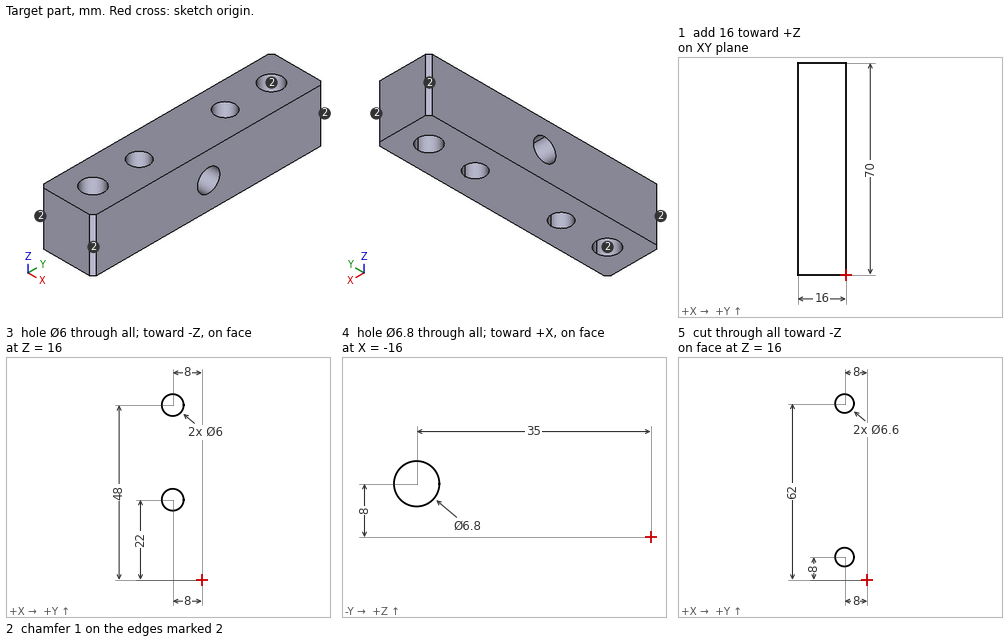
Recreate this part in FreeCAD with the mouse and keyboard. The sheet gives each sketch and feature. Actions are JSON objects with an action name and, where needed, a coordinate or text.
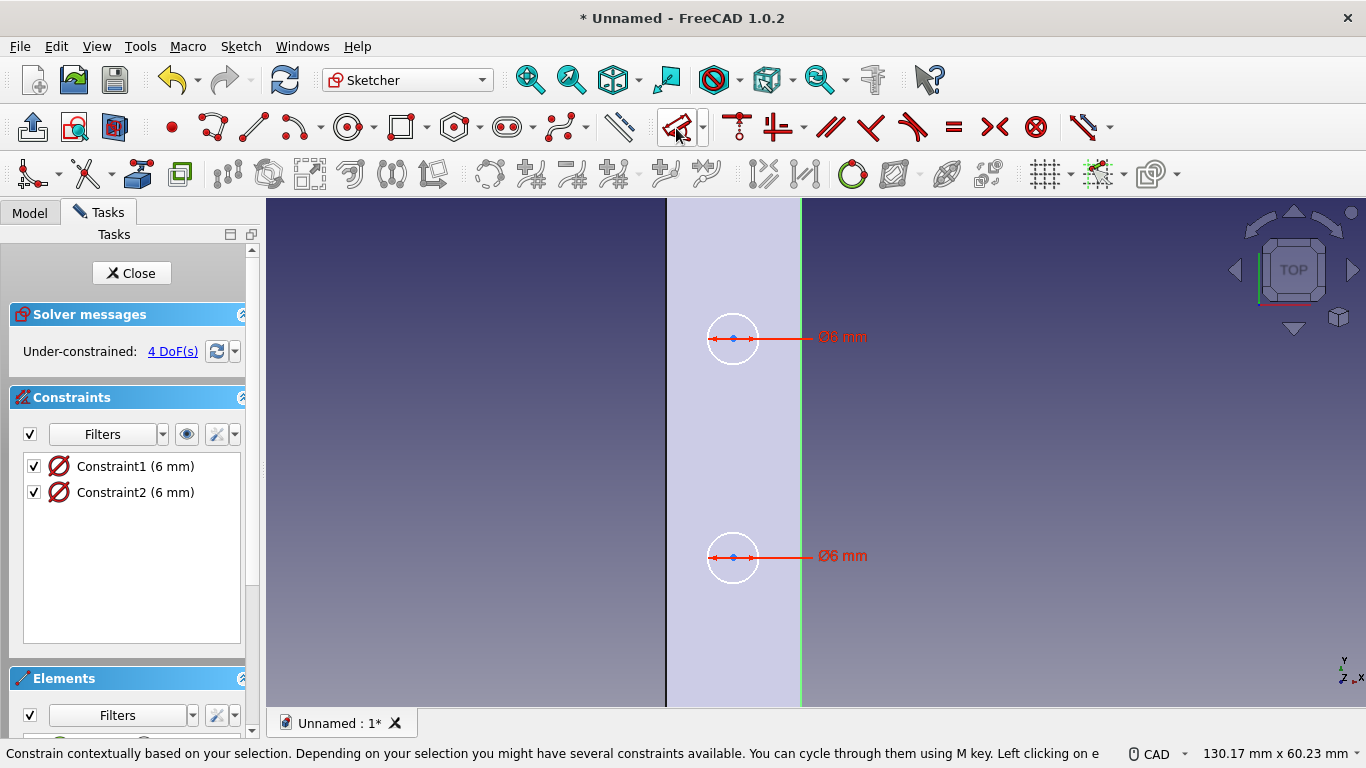
{"action": "left_click", "coordinate": [733, 339]}
{"action": "left_click", "coordinate": [767, 305]}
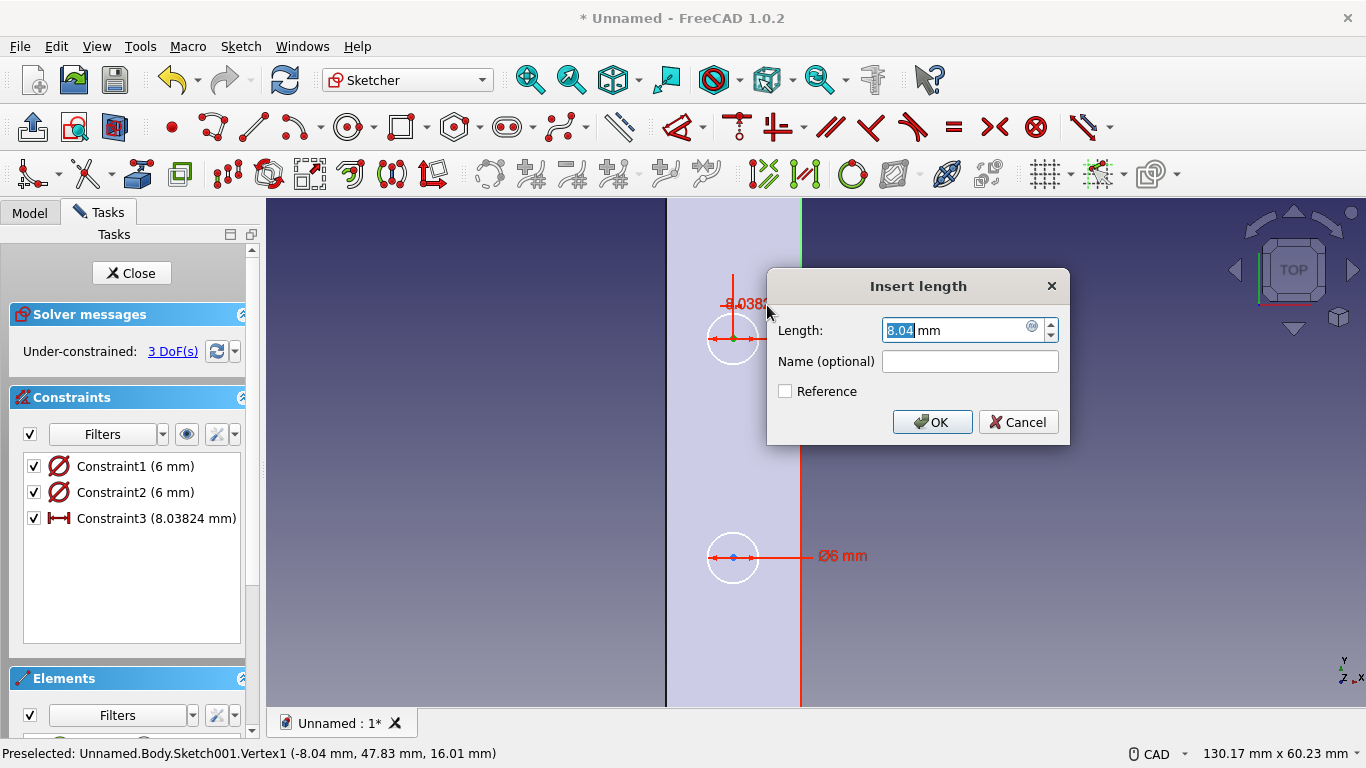
{"action": "type", "text": "8"}
{"action": "key", "text": "Return"}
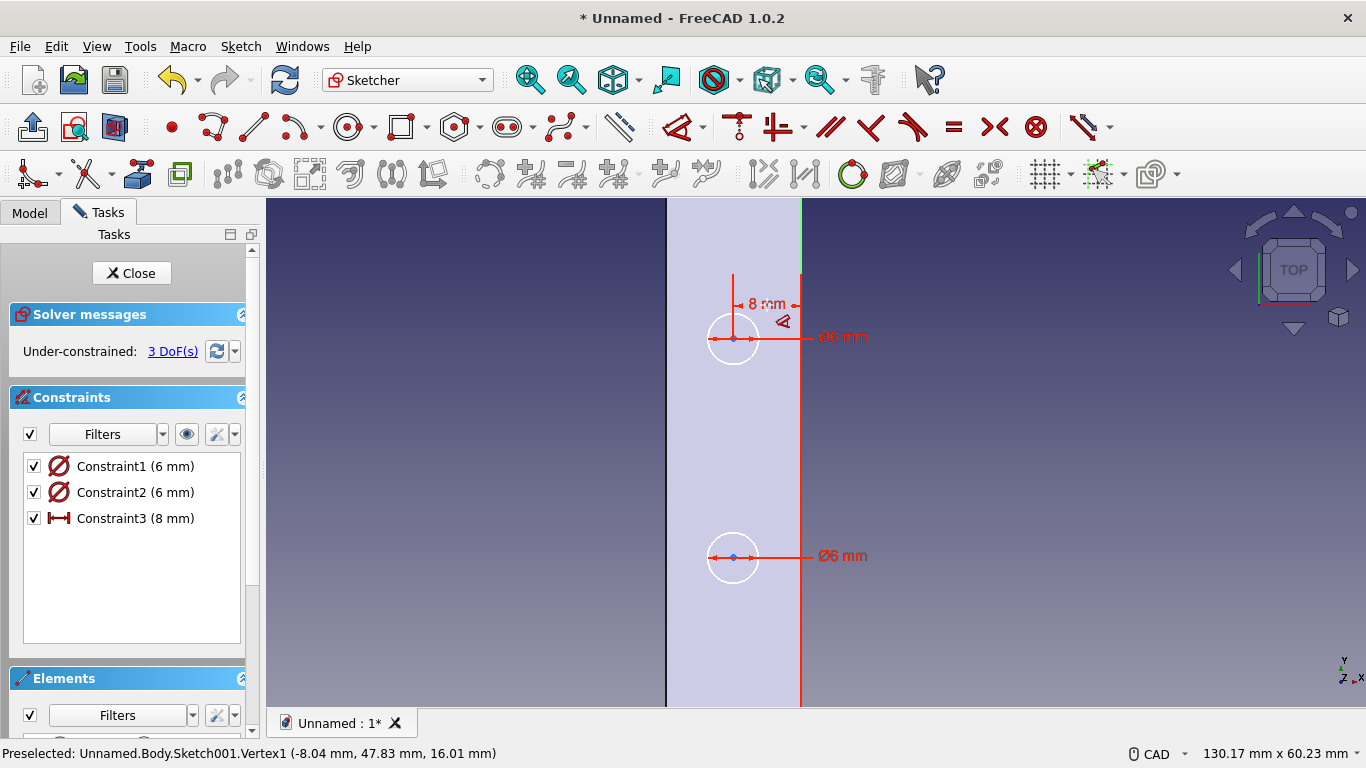
{"action": "left_click", "coordinate": [733, 558]}
{"action": "left_click", "coordinate": [767, 524]}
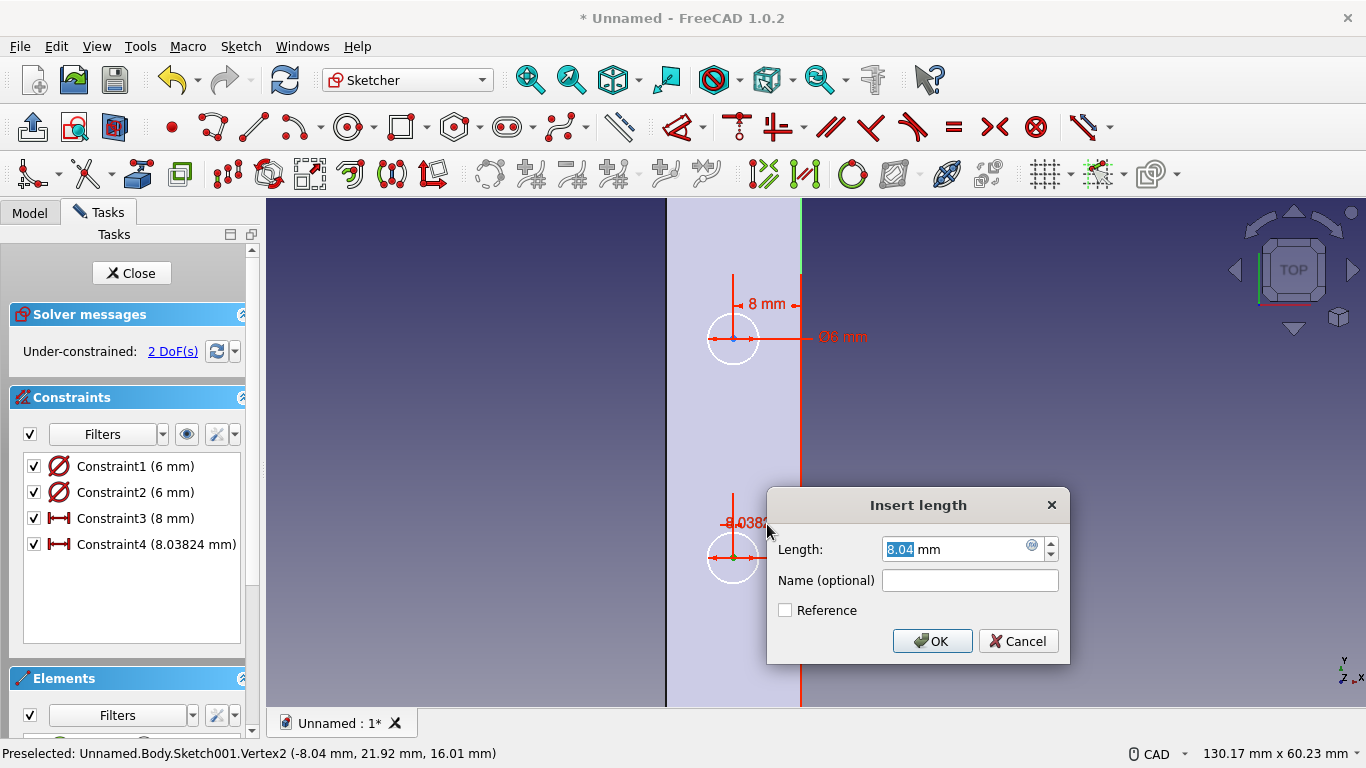
{"action": "type", "text": "8"}
{"action": "key", "text": "Return"}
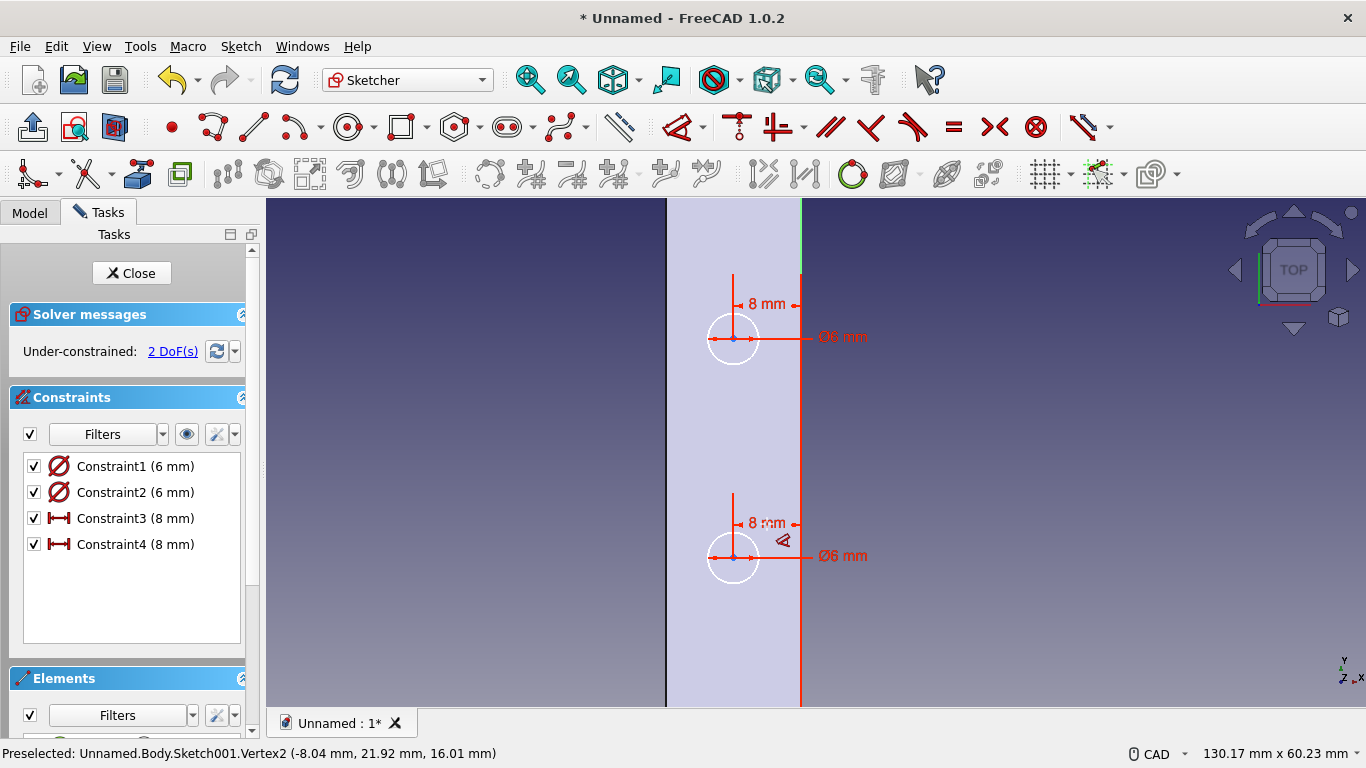
{"action": "left_click", "coordinate": [733, 339]}
{"action": "left_click", "coordinate": [835, 431]}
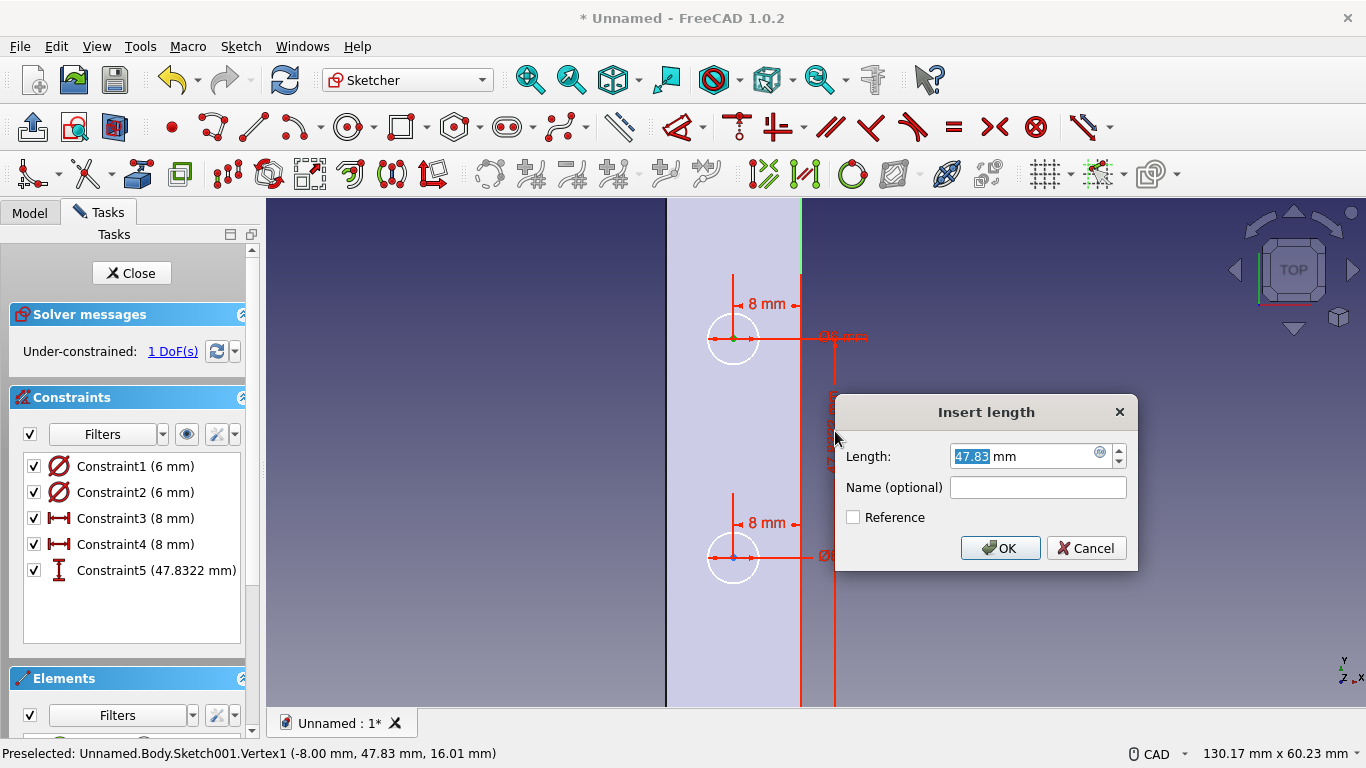
{"action": "type", "text": "48"}
{"action": "key", "text": "Return"}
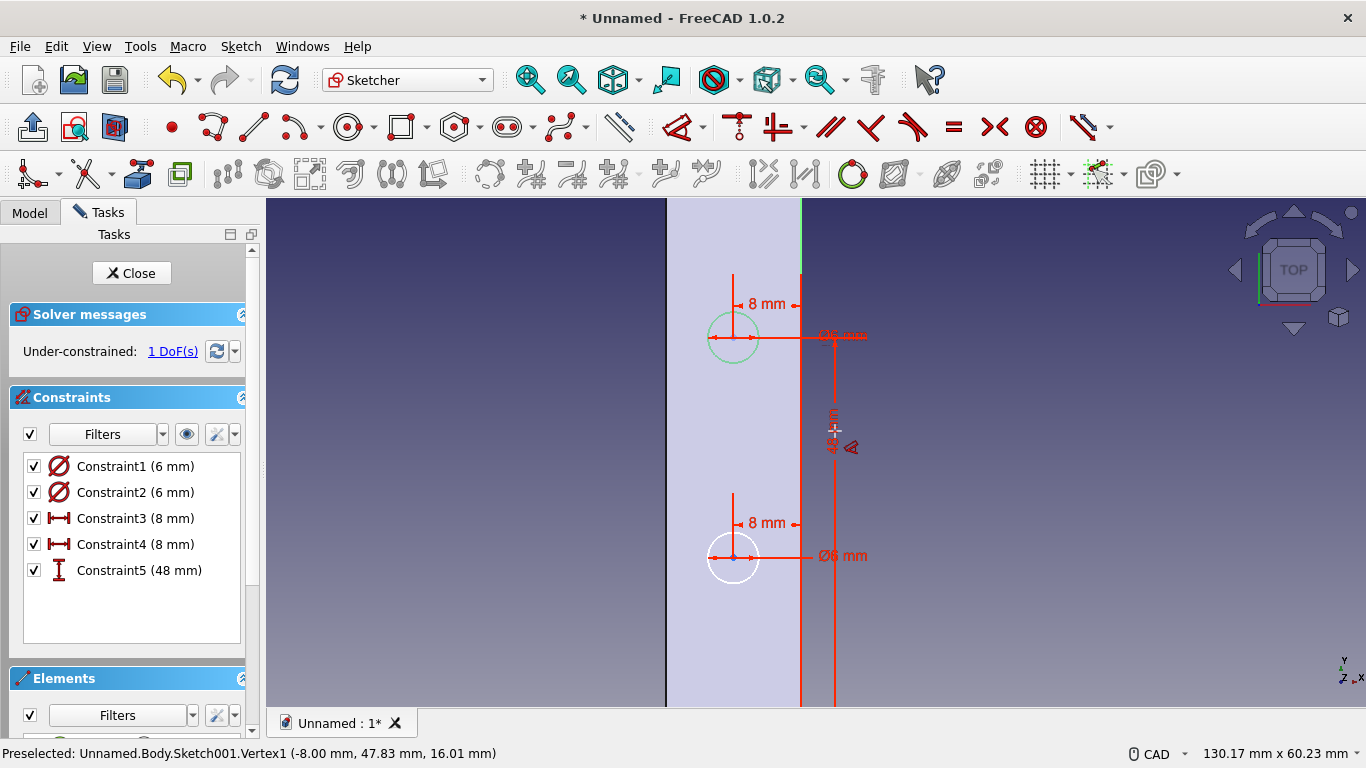
{"action": "left_click", "coordinate": [733, 558]}
{"action": "left_click", "coordinate": [835, 619]}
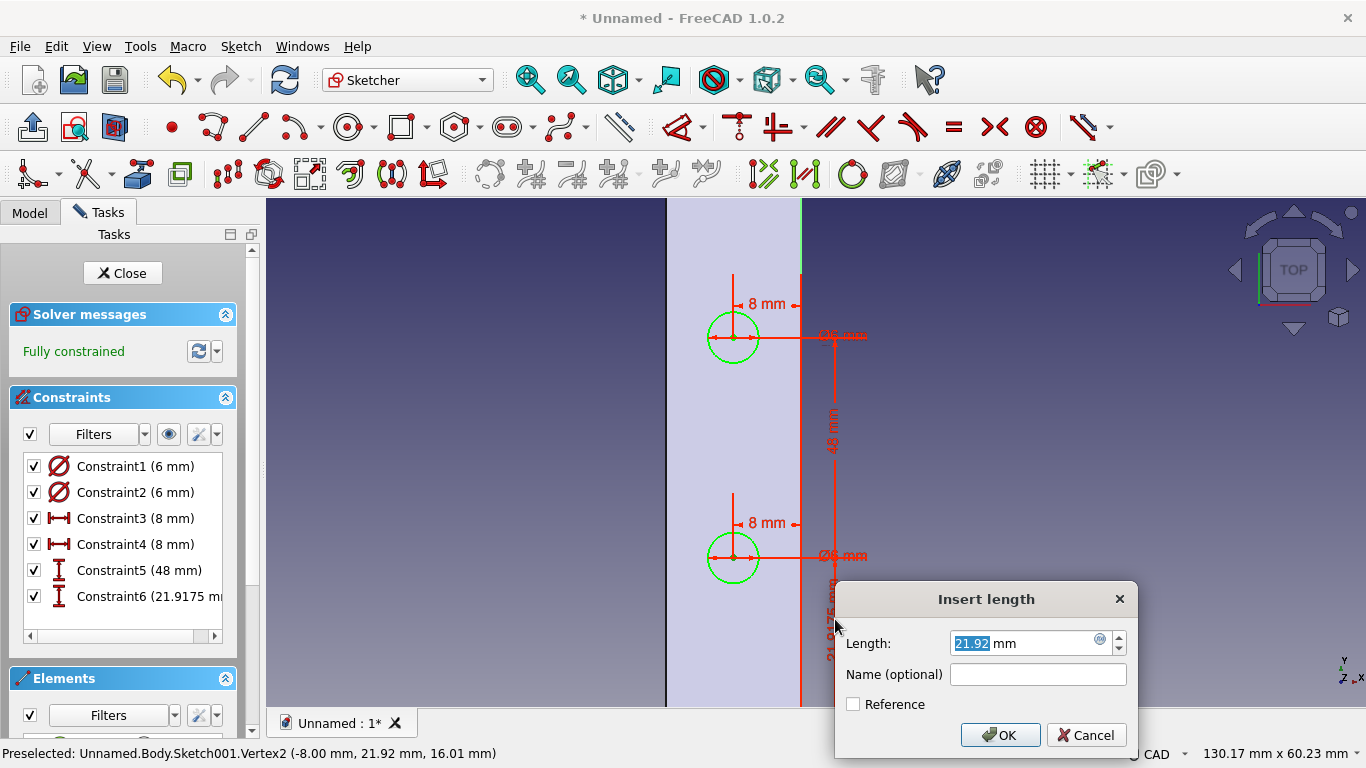
{"action": "type", "text": "22"}
{"action": "key", "text": "Return"}
{"action": "key", "text": "Escape"}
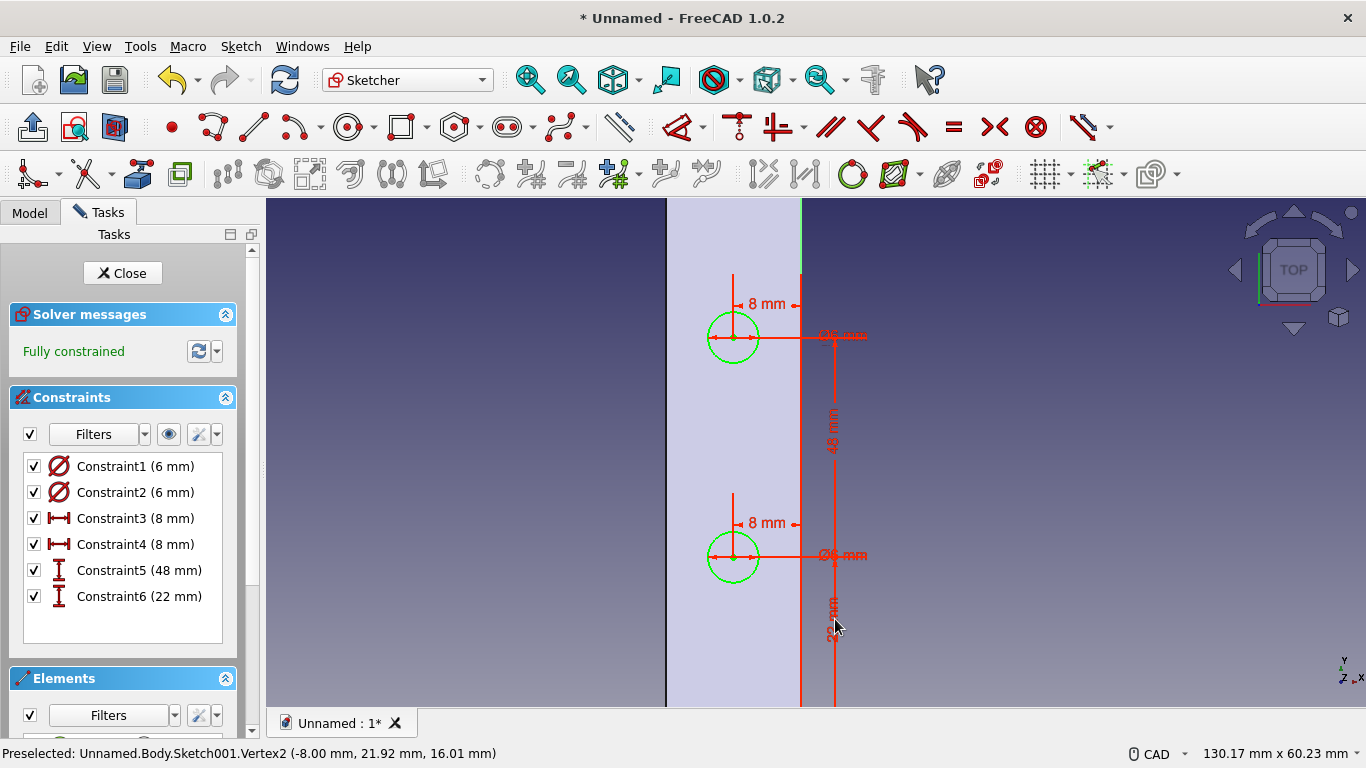
{"action": "left_click", "coordinate": [123, 273]}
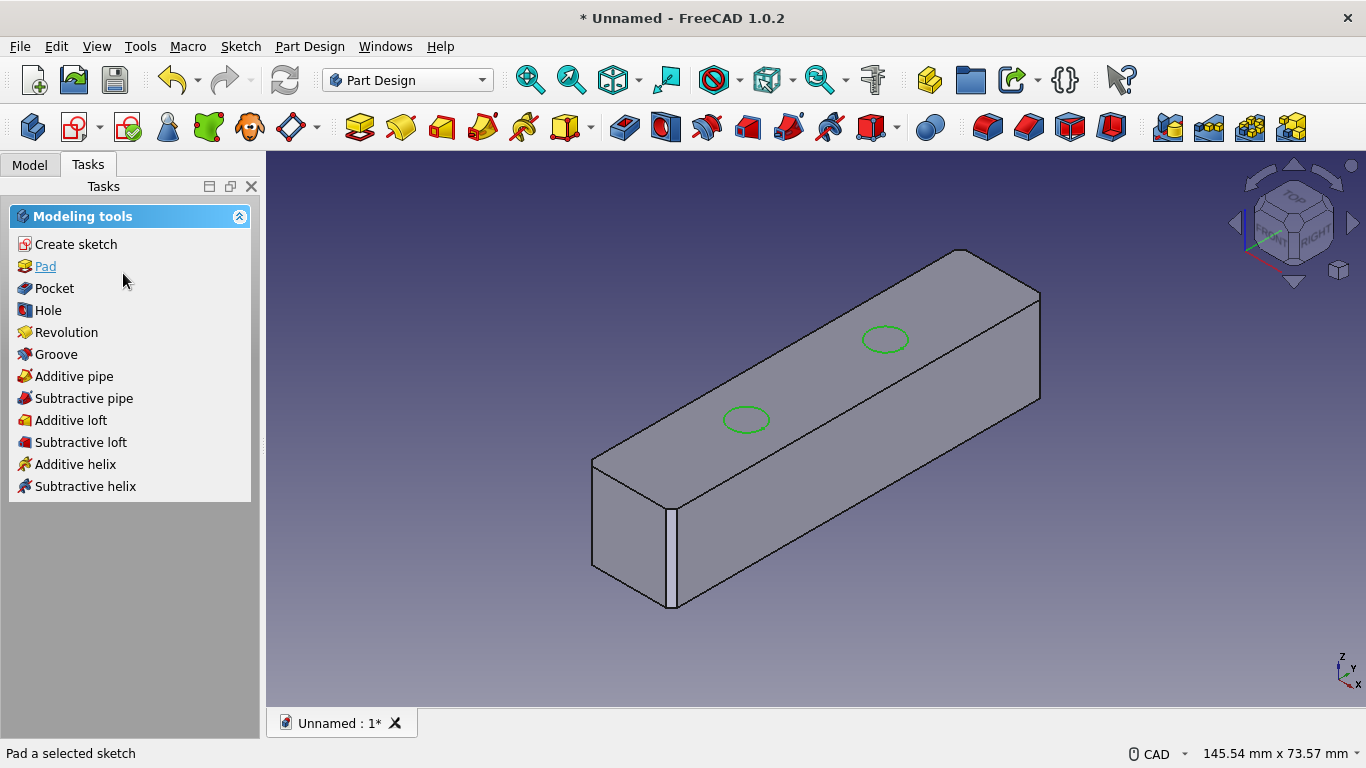
{"action": "left_click", "coordinate": [666, 128]}